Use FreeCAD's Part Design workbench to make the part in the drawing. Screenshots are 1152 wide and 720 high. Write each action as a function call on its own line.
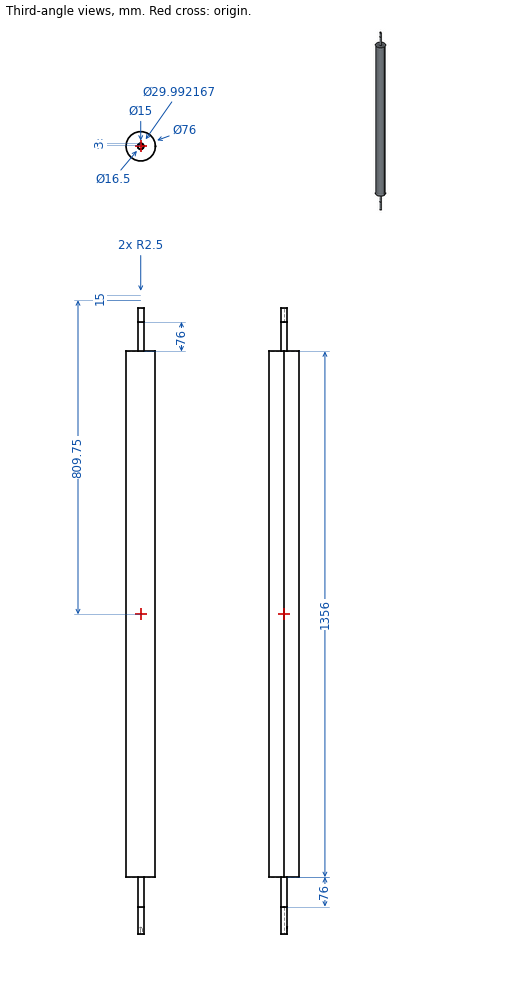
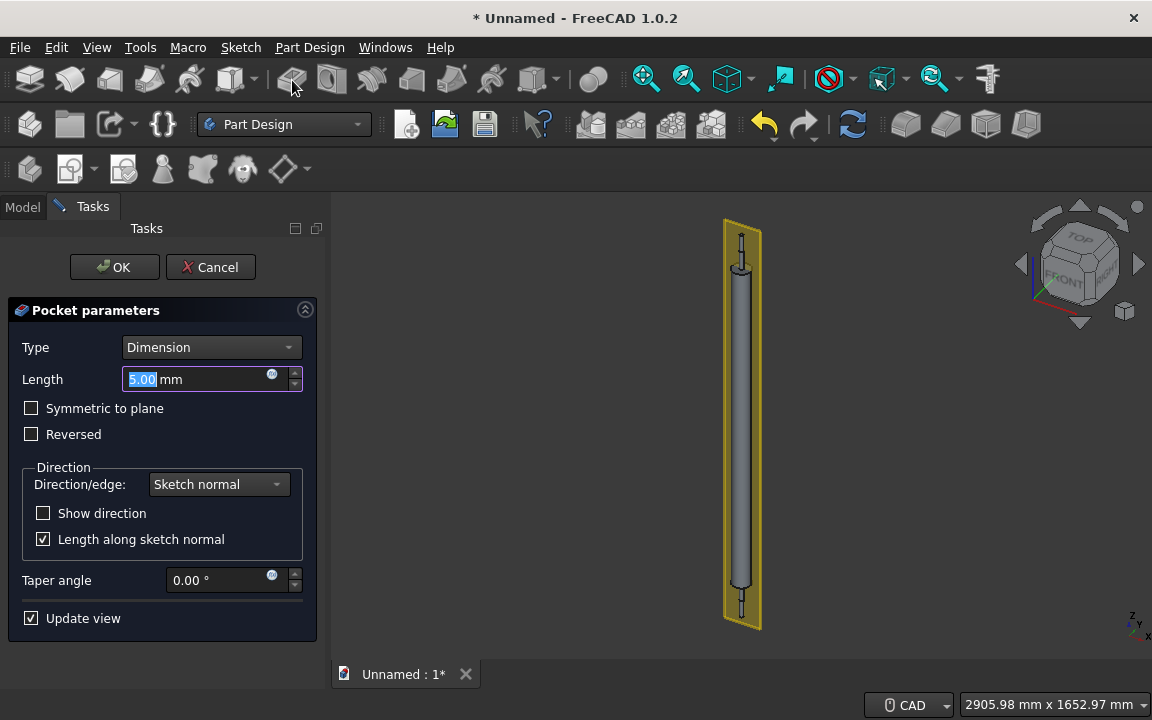
text(3)
key(Tab)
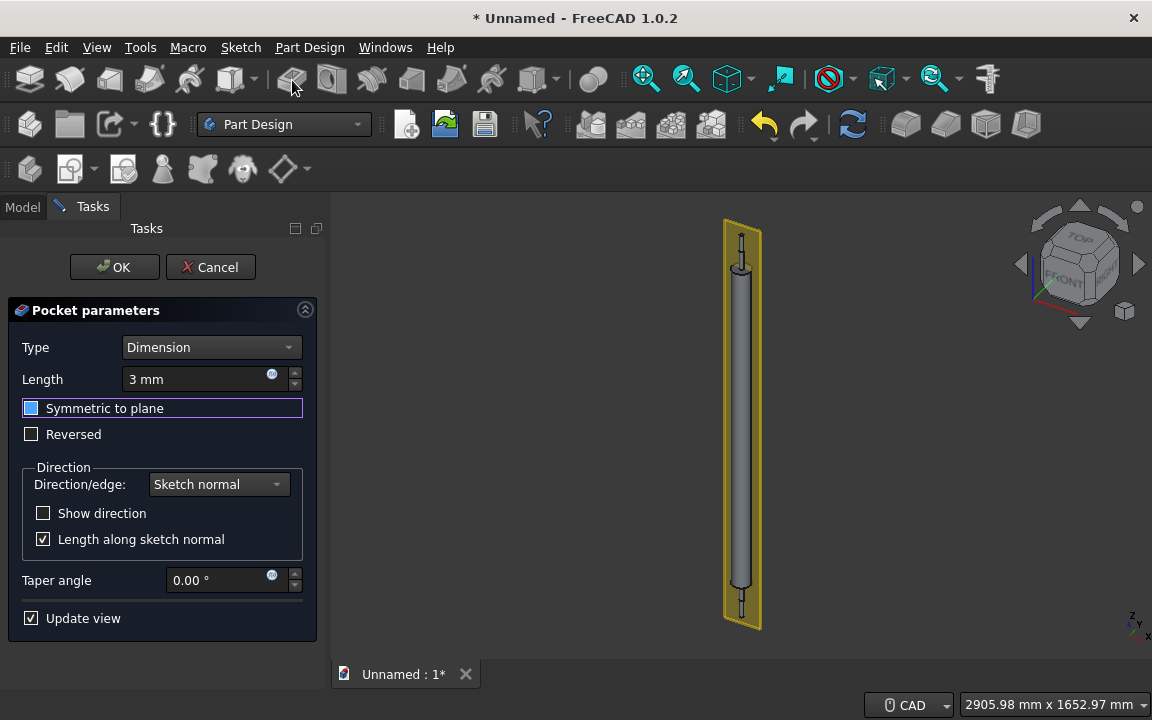
click(30, 434)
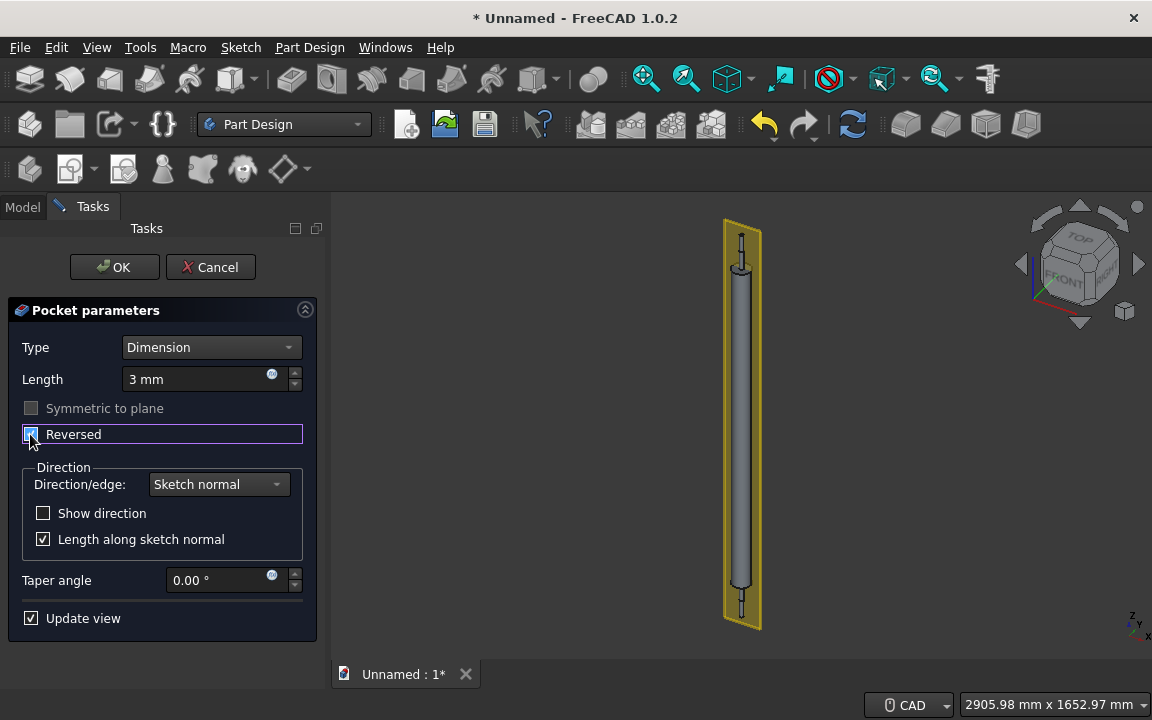
click(115, 267)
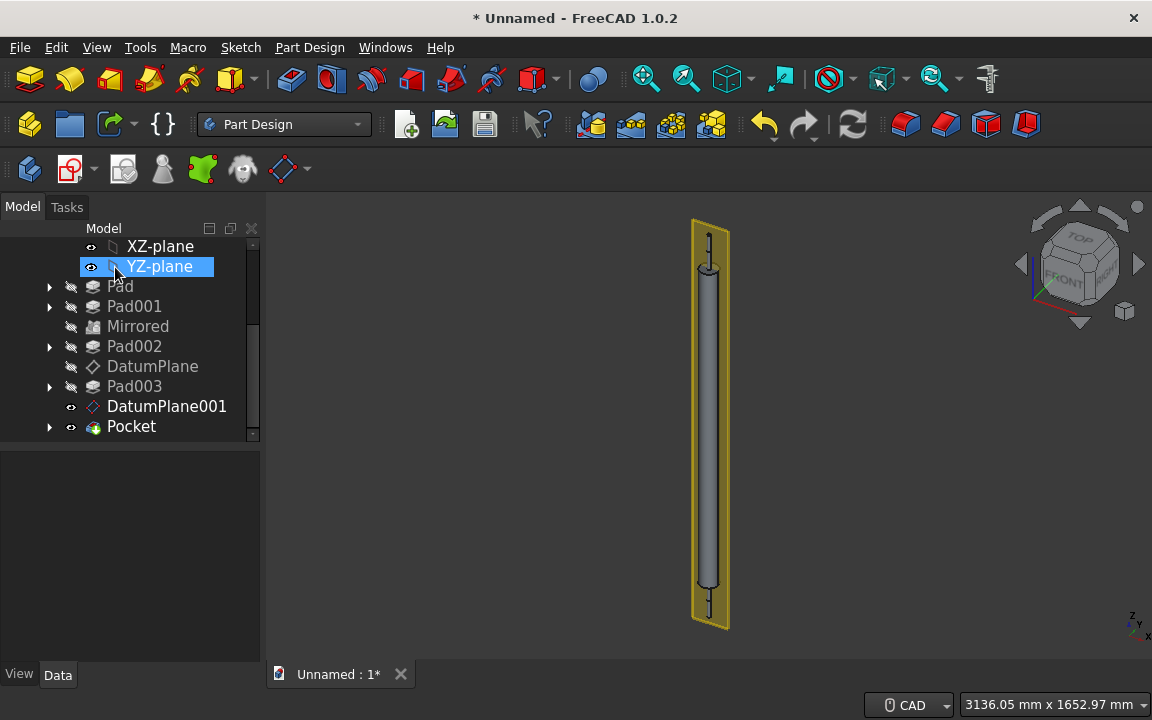
click(116, 407)
key(space)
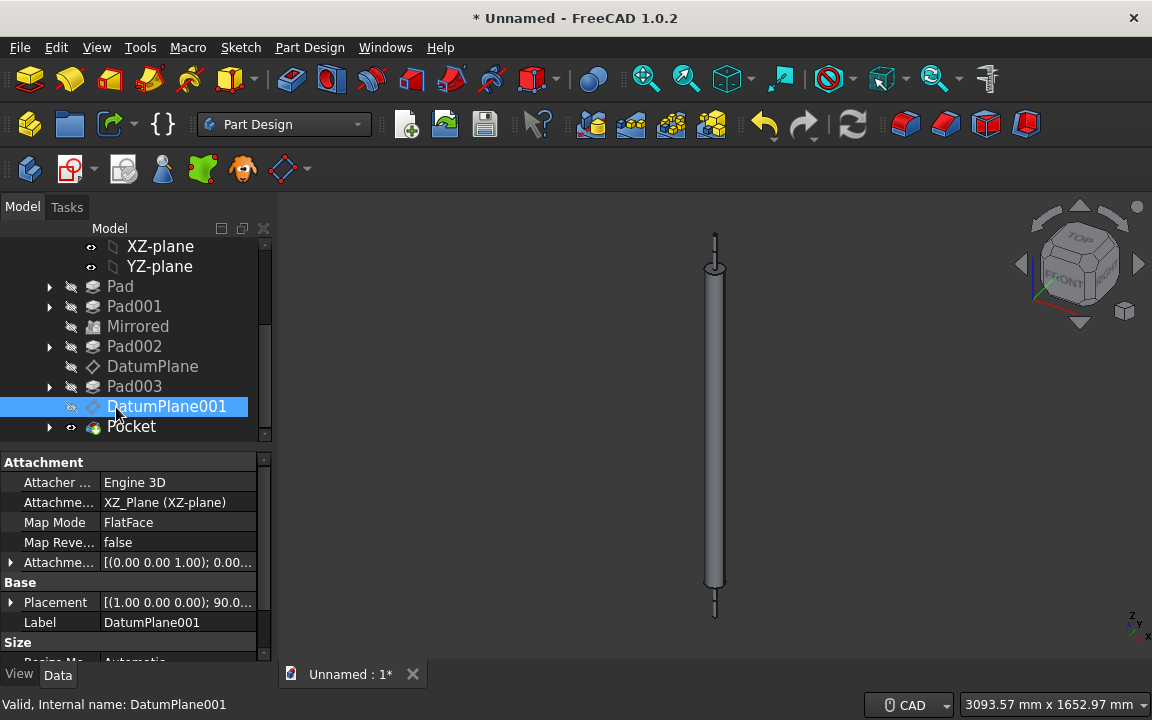
click(116, 427)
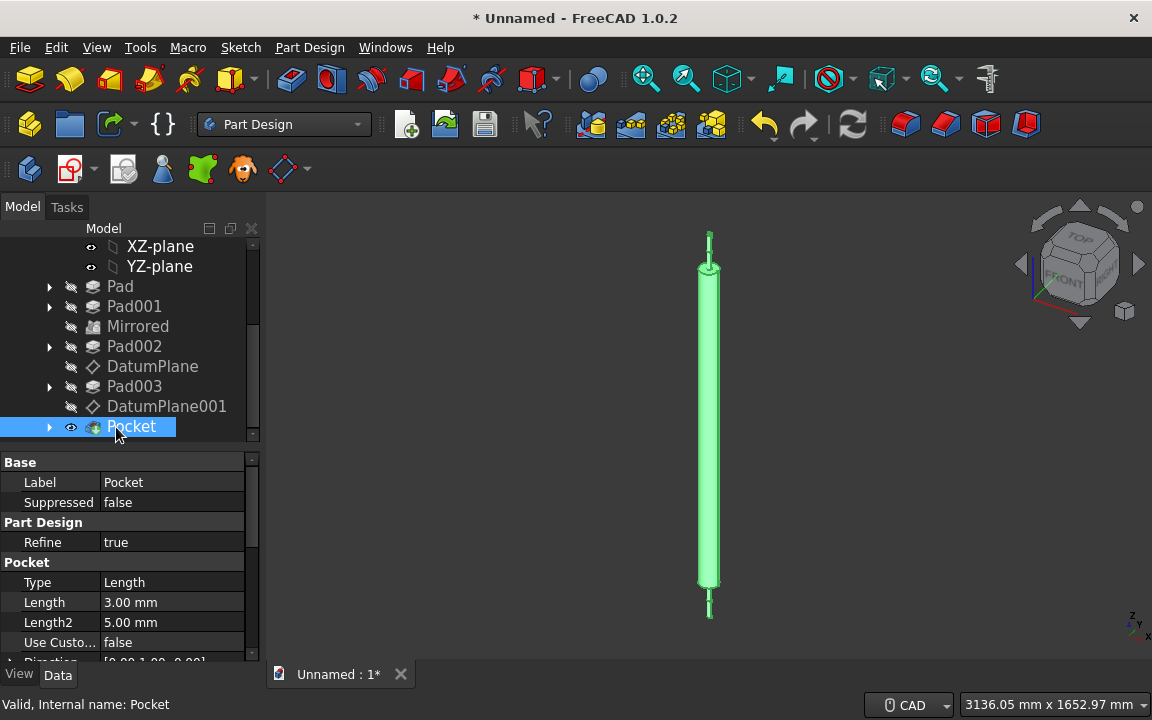
click(592, 124)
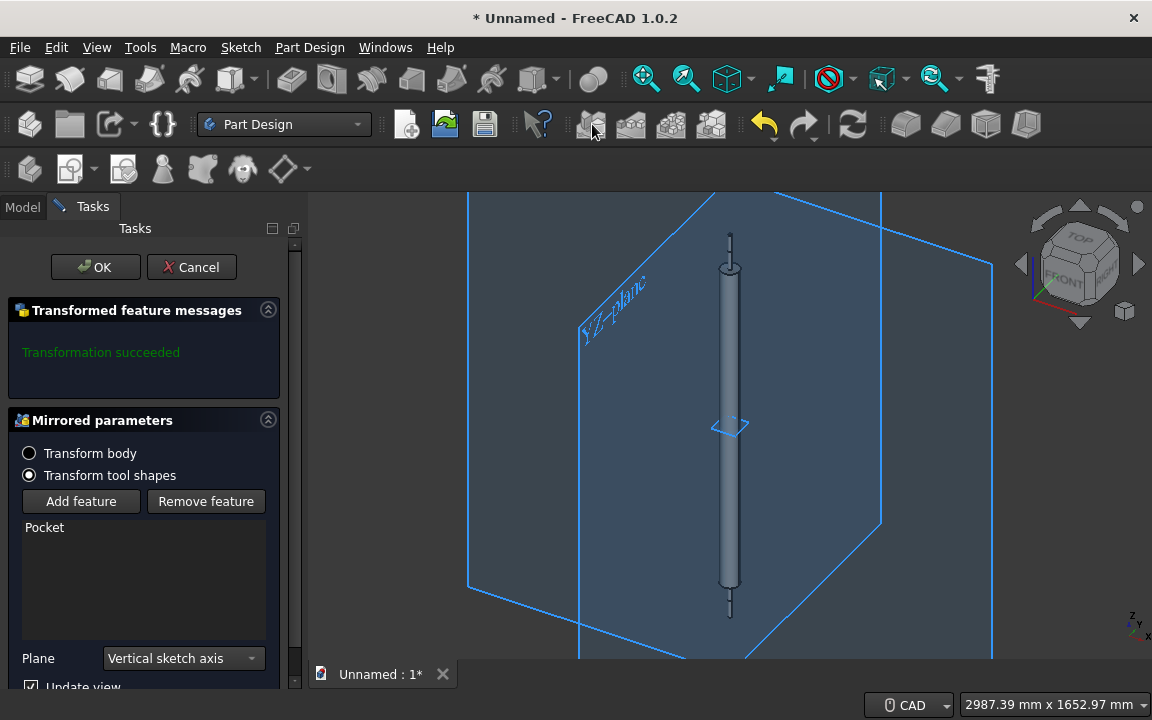
click(184, 658)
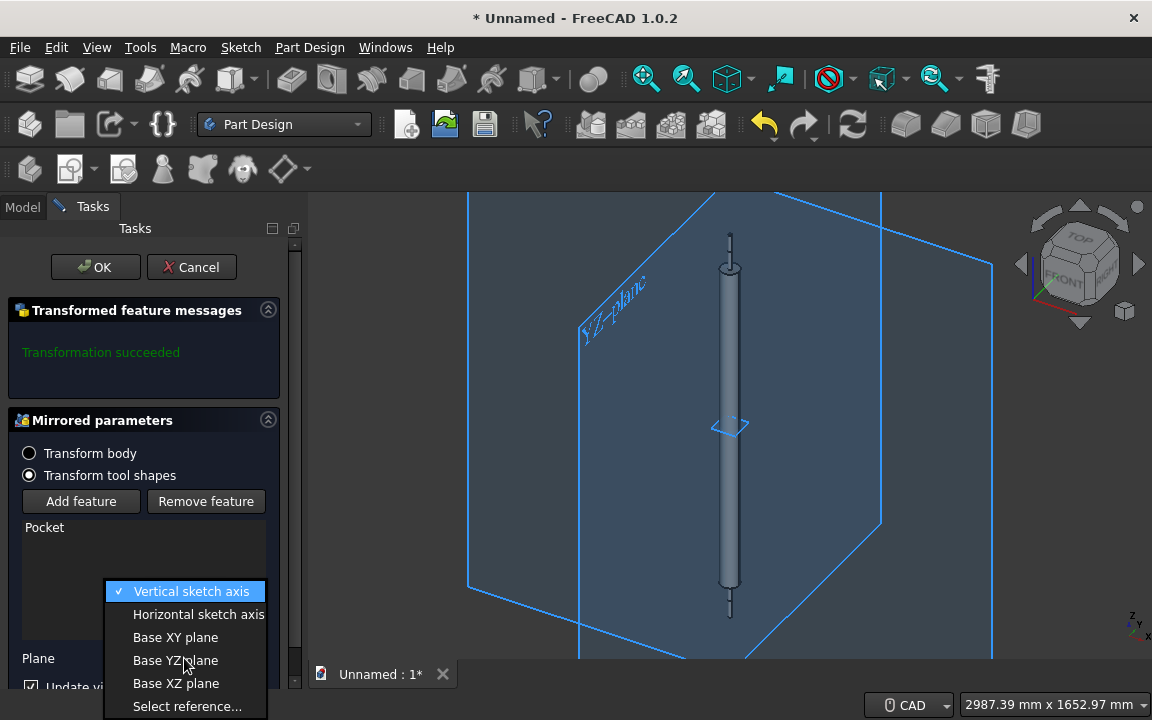
click(184, 638)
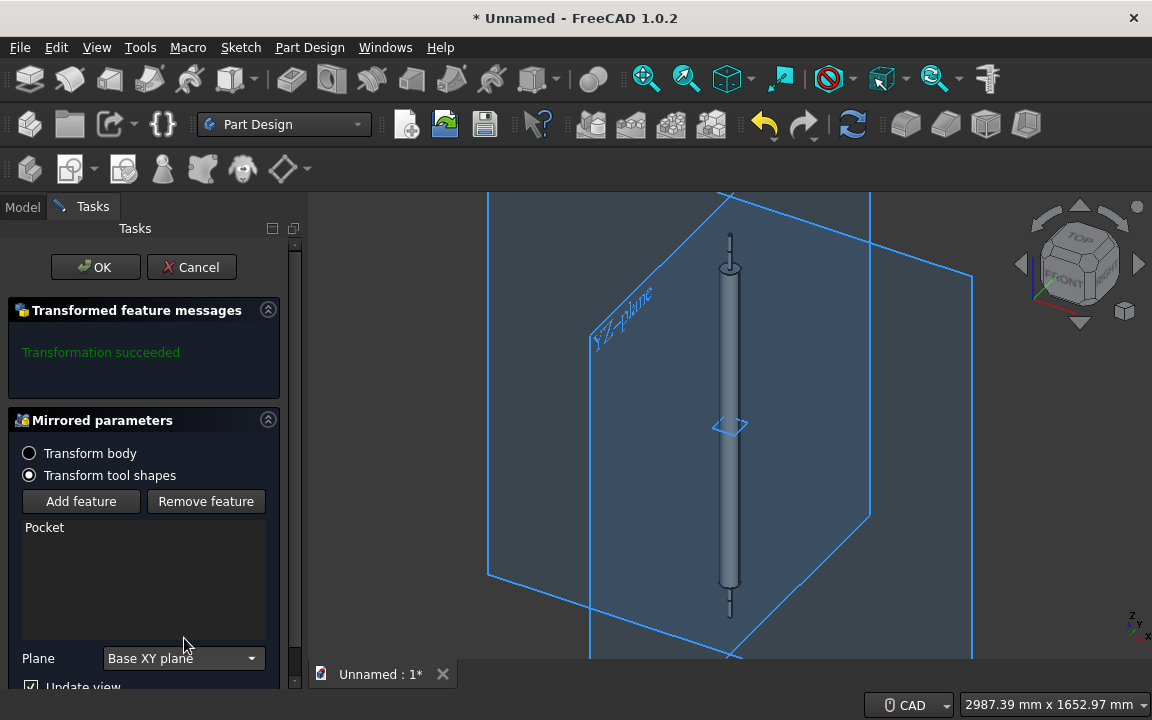
click(96, 267)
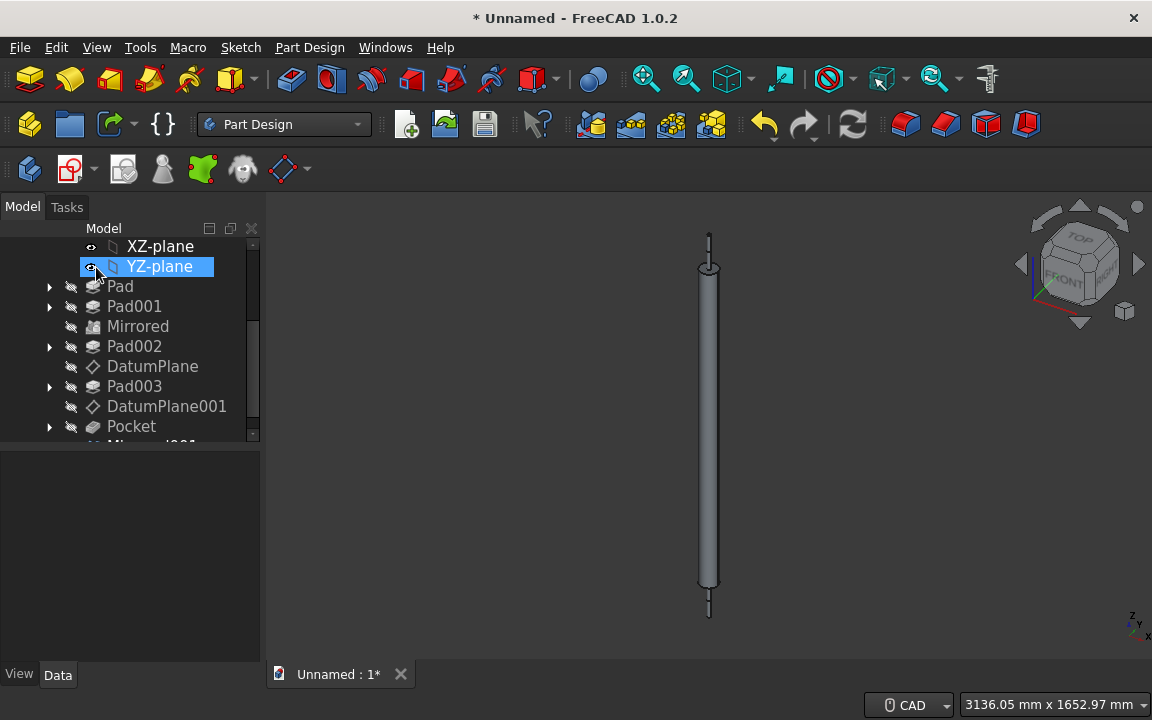
scroll(709, 234, up, 11)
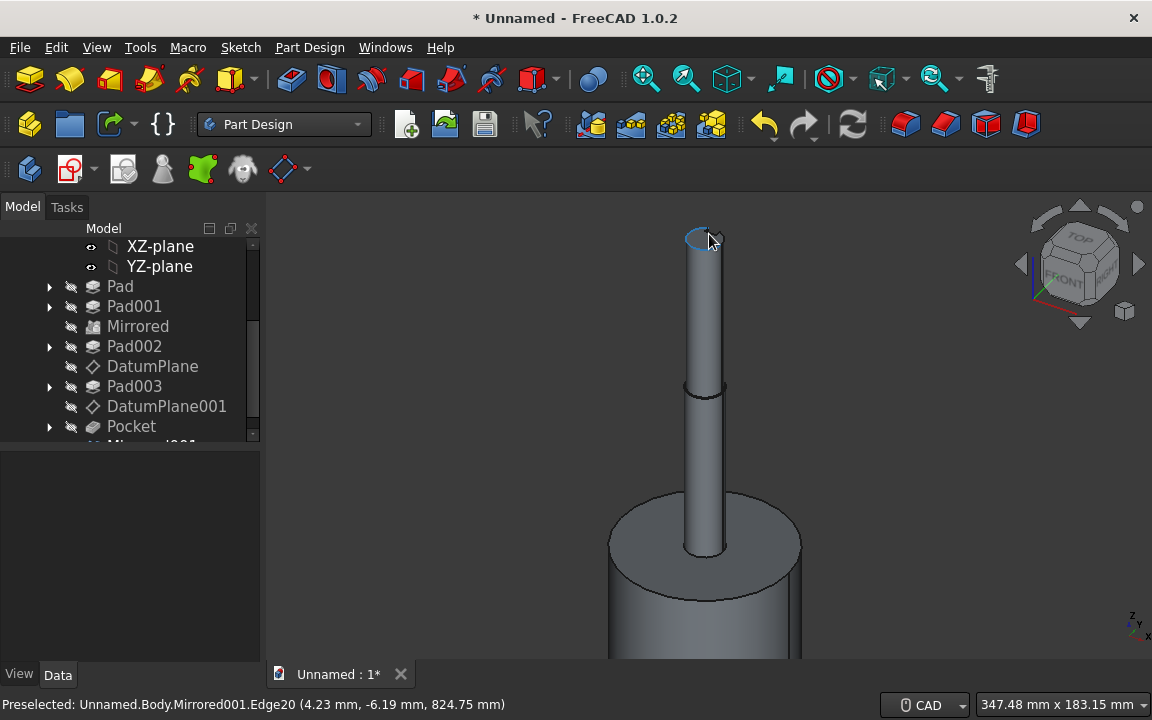
click(705, 238)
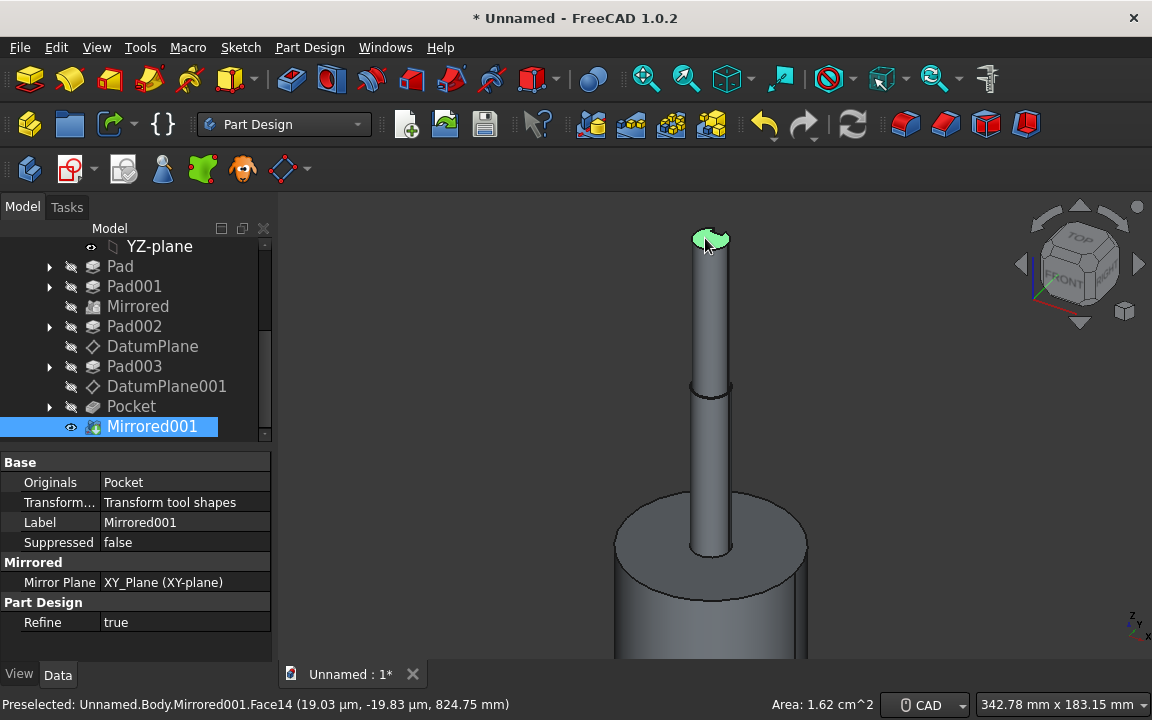
click(70, 170)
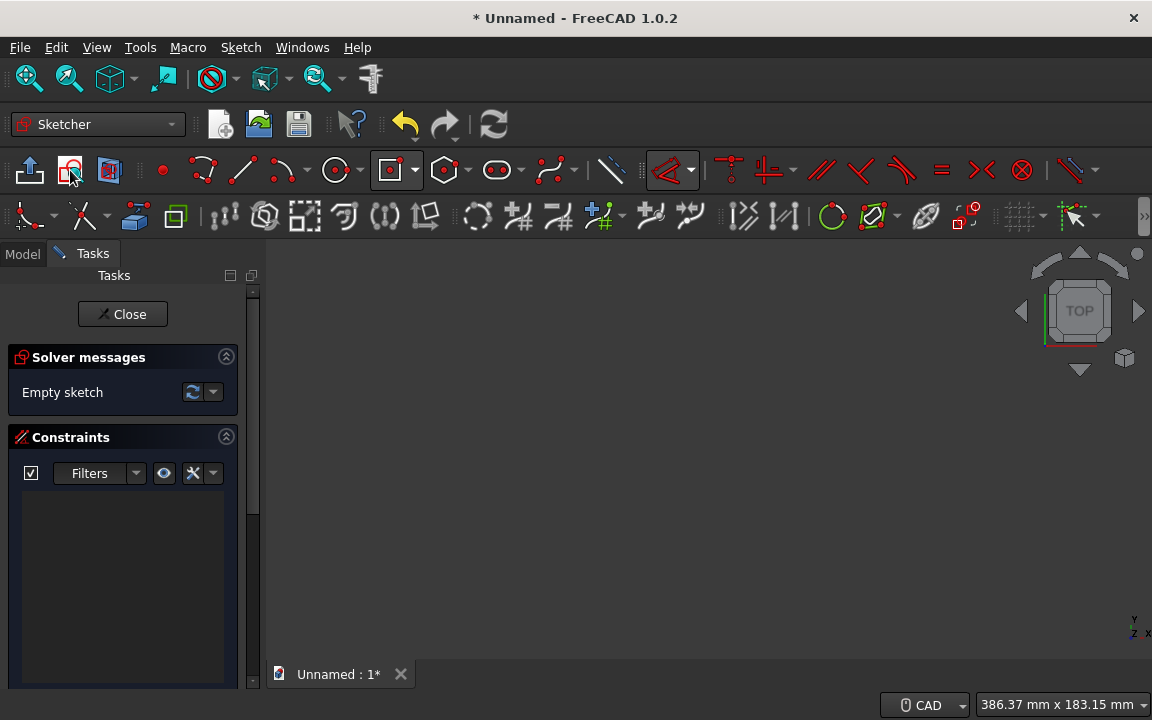
scroll(640, 449, down, 5)